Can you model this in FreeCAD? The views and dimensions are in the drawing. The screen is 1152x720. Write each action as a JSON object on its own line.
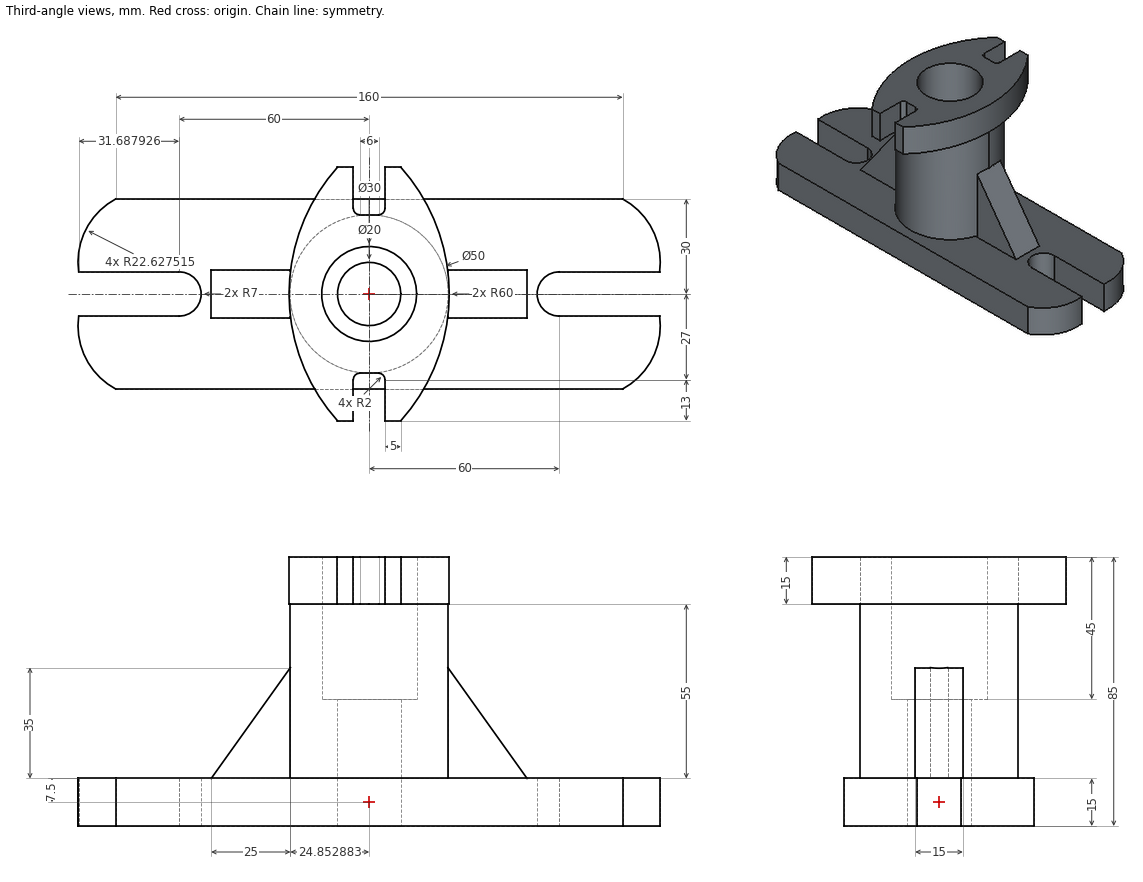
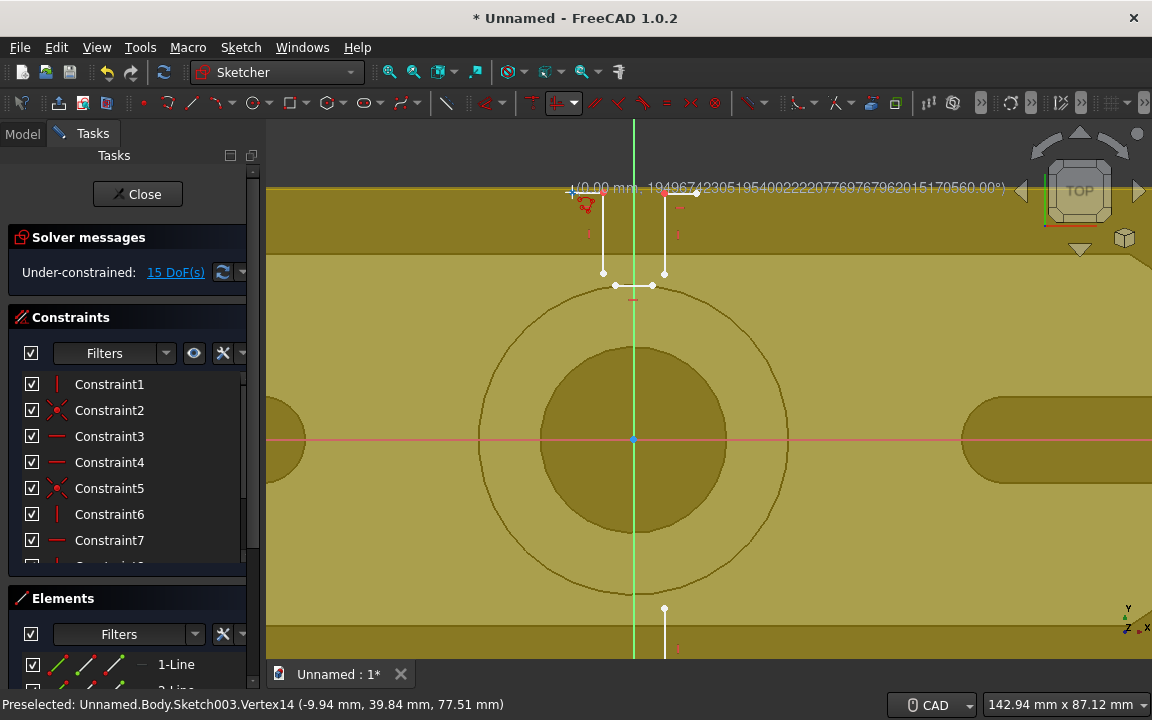
{"action": "scroll", "coordinate": [655, 285], "scroll_direction": "down", "scroll_amount": 2}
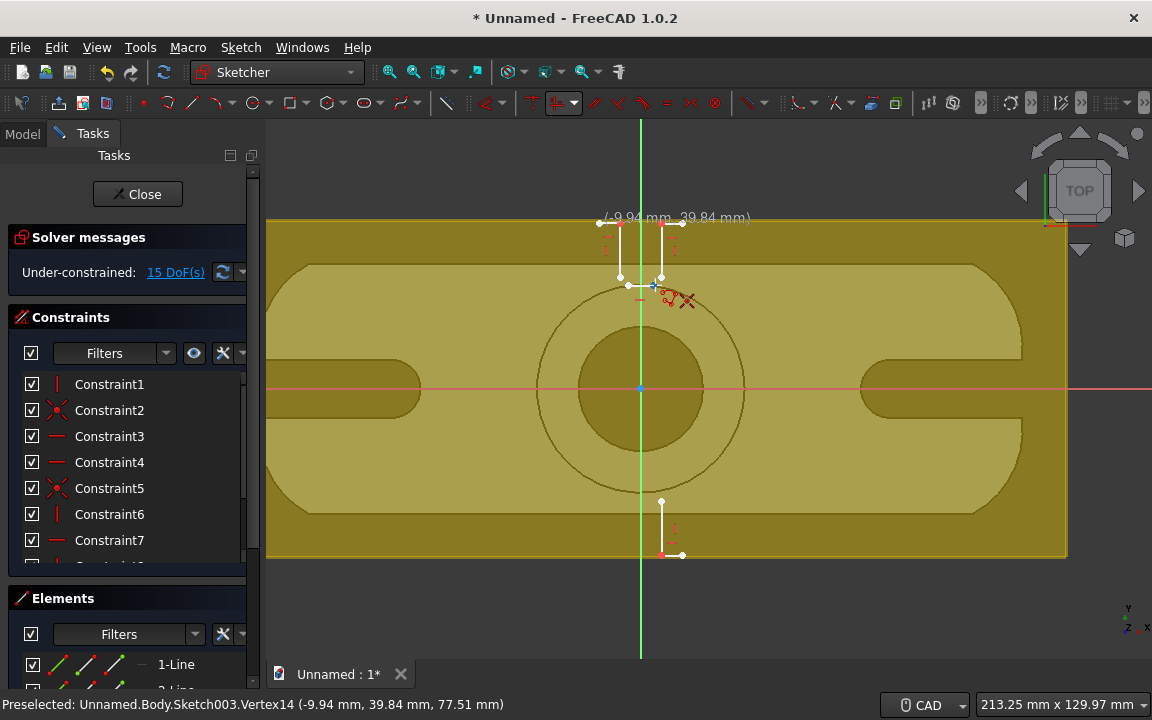
{"action": "left_click", "coordinate": [599, 555]}
{"action": "left_click", "coordinate": [620, 555]}
{"action": "left_click", "coordinate": [620, 501]}
{"action": "right_click", "coordinate": [620, 501]}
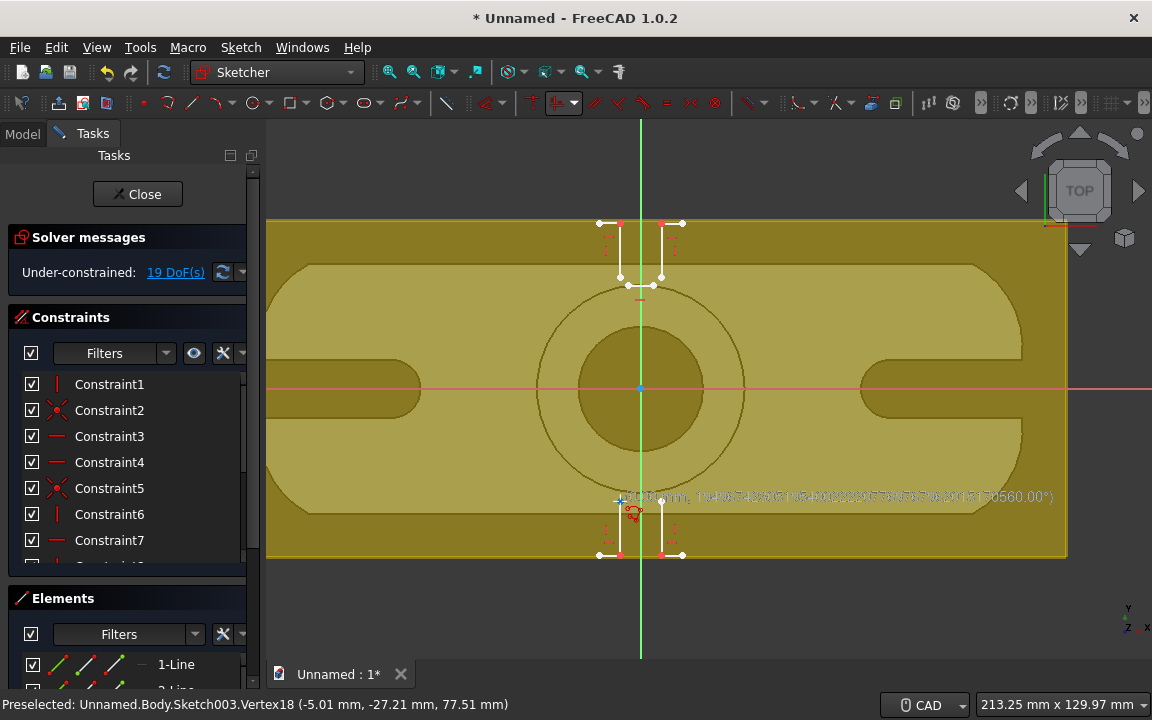
{"action": "key", "text": "g l"}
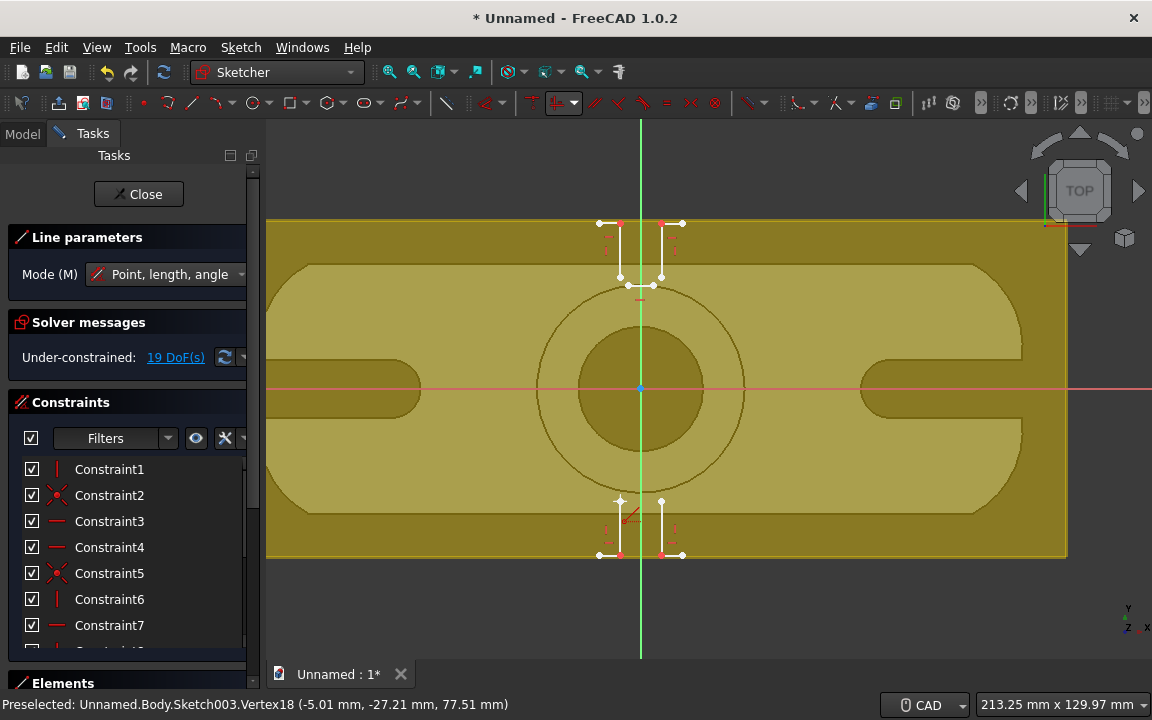
{"action": "scroll", "coordinate": [628, 493], "scroll_direction": "up", "scroll_amount": 2}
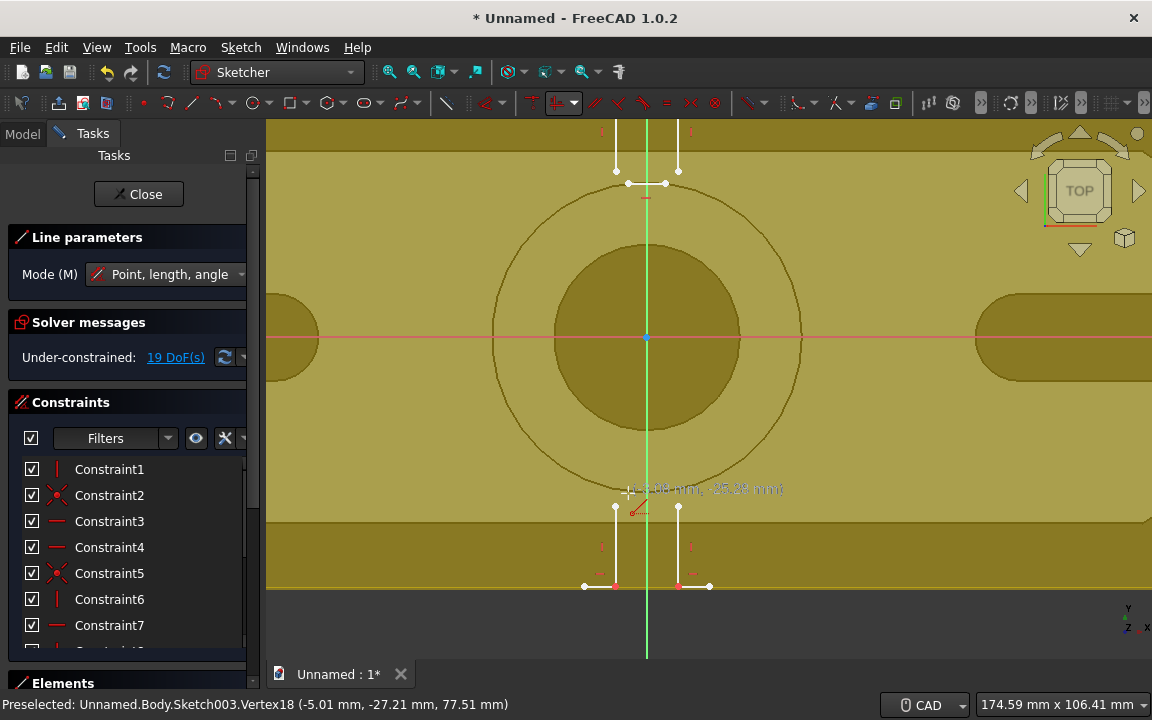
{"action": "left_click", "coordinate": [628, 492]}
{"action": "left_click", "coordinate": [665, 492]}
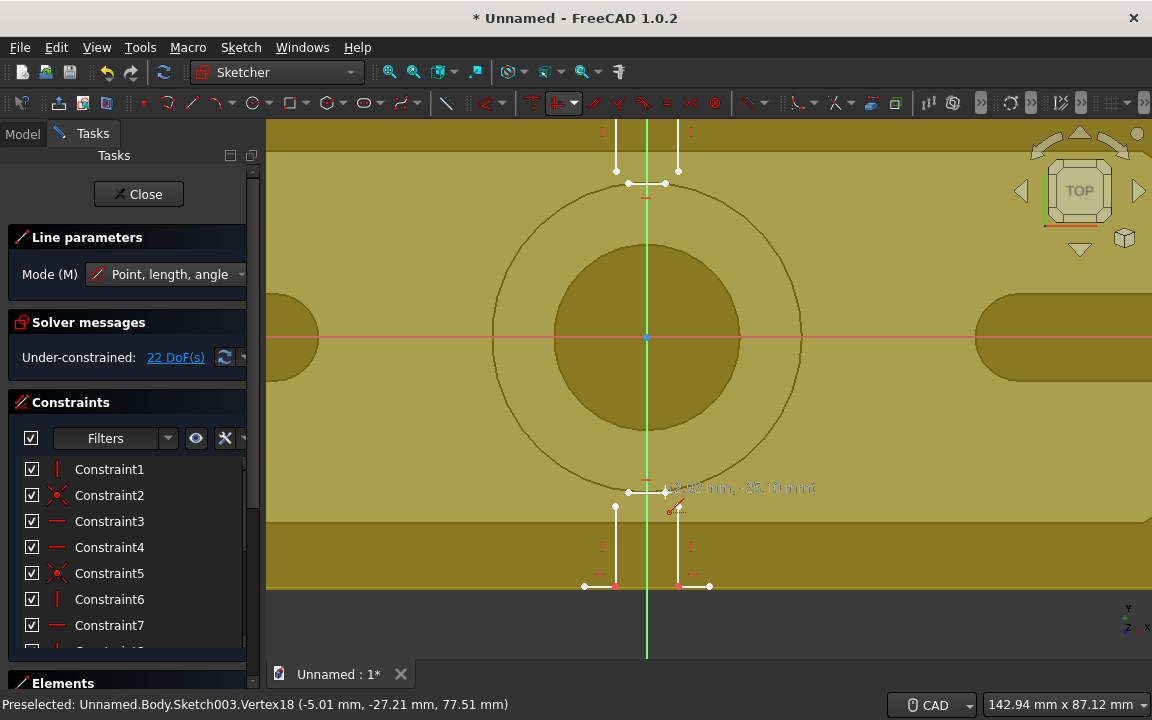
{"action": "key", "text": "g 3 a"}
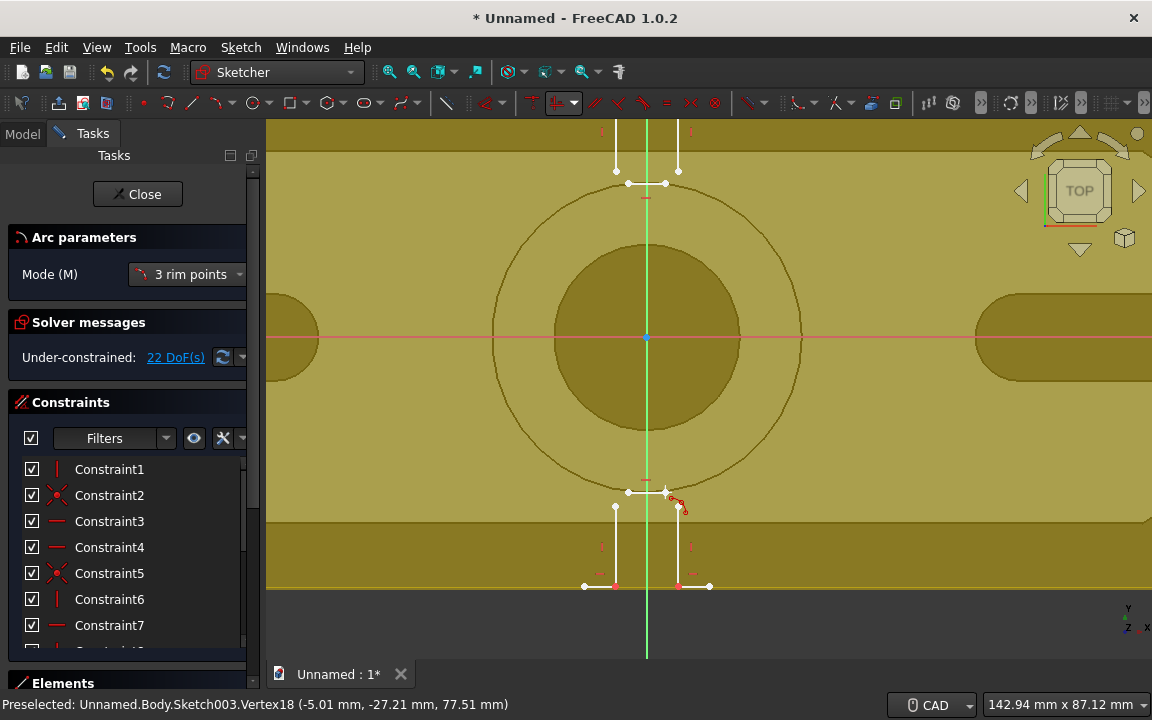
{"action": "left_click", "coordinate": [709, 587]}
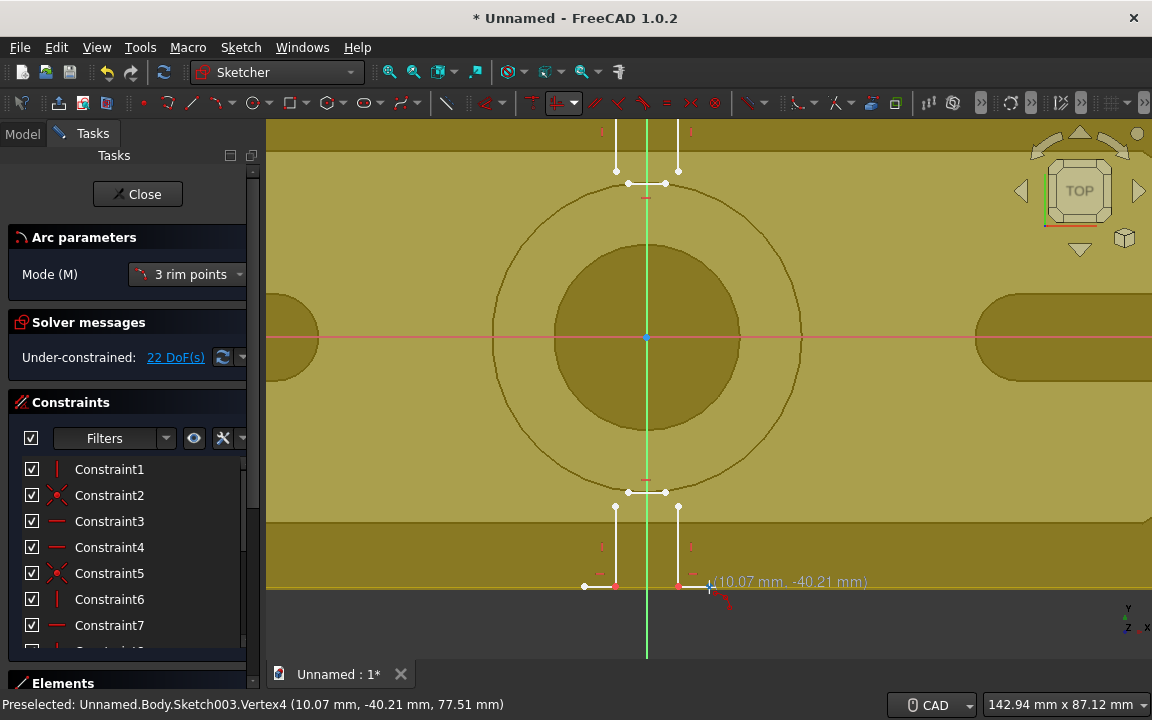
{"action": "scroll", "coordinate": [627, 494], "scroll_direction": "down", "scroll_amount": 2}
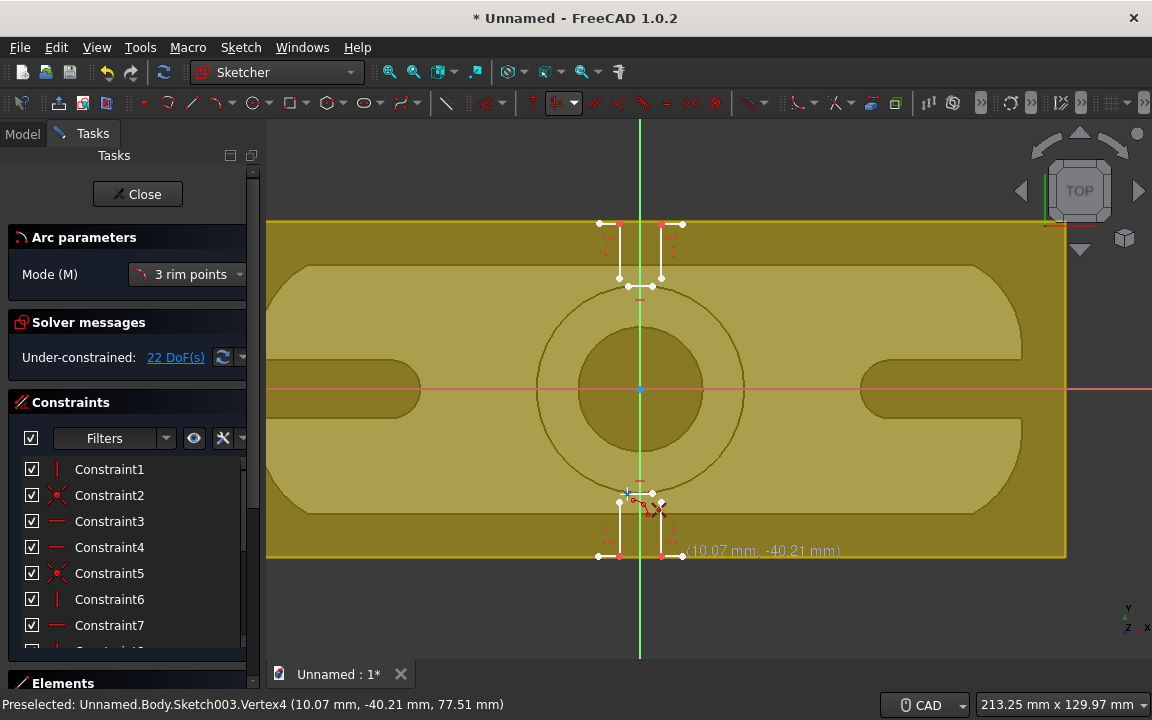
{"action": "scroll", "coordinate": [682, 223], "scroll_direction": "up", "scroll_amount": 3}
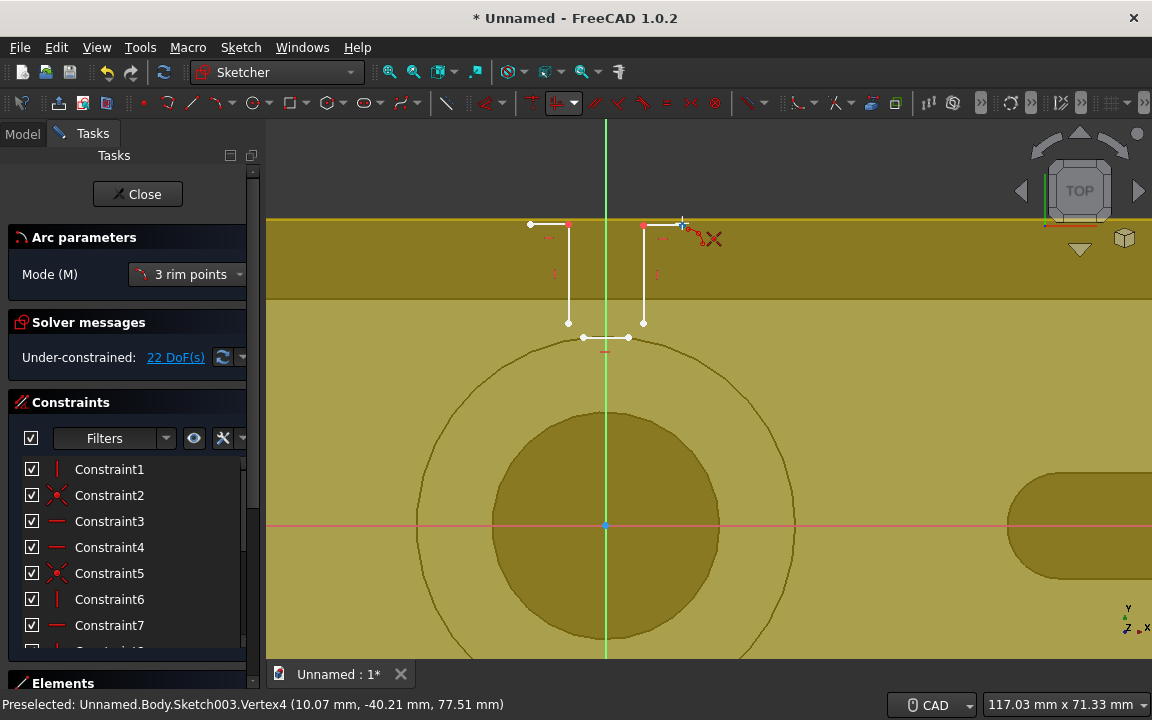
{"action": "left_click", "coordinate": [682, 225]}
{"action": "left_click", "coordinate": [792, 592]}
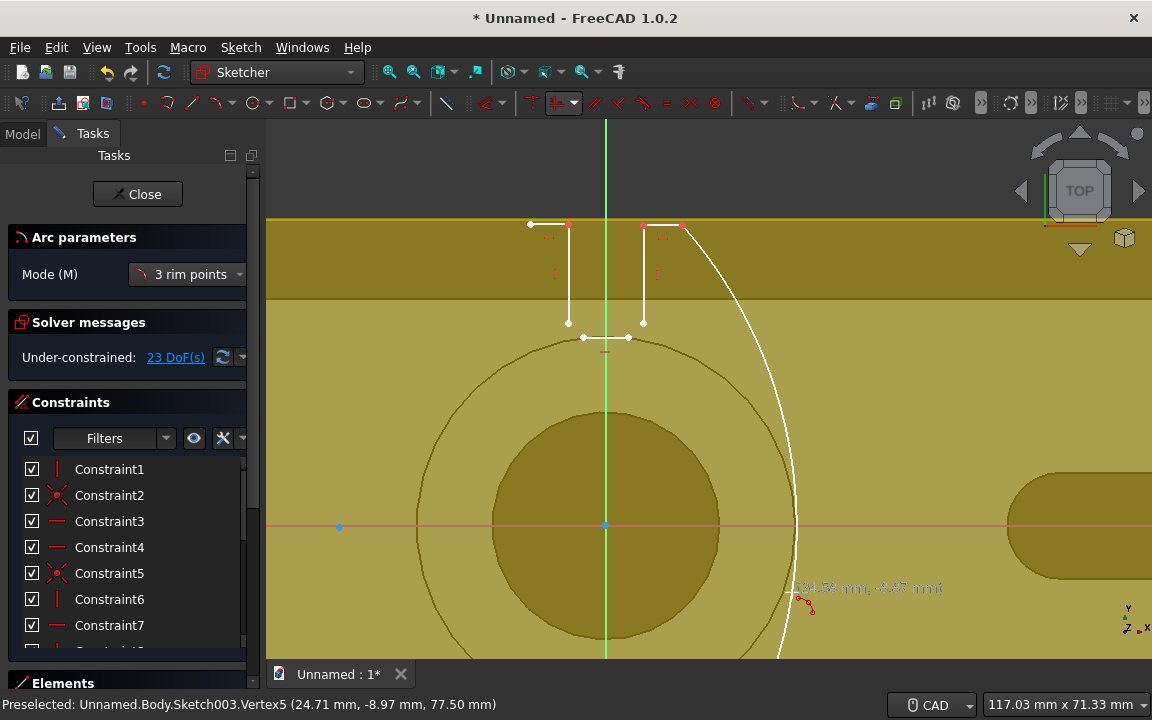
{"action": "left_click", "coordinate": [644, 324]}
{"action": "left_click", "coordinate": [628, 338]}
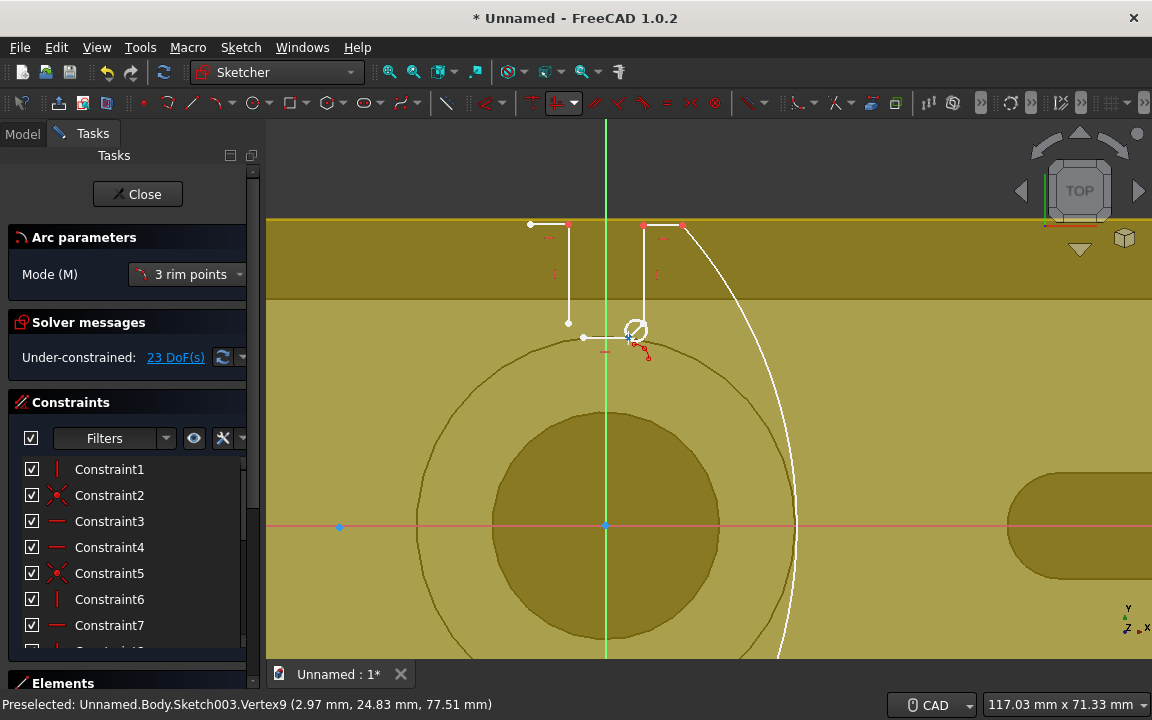
{"action": "scroll", "coordinate": [639, 332], "scroll_direction": "up", "scroll_amount": 7}